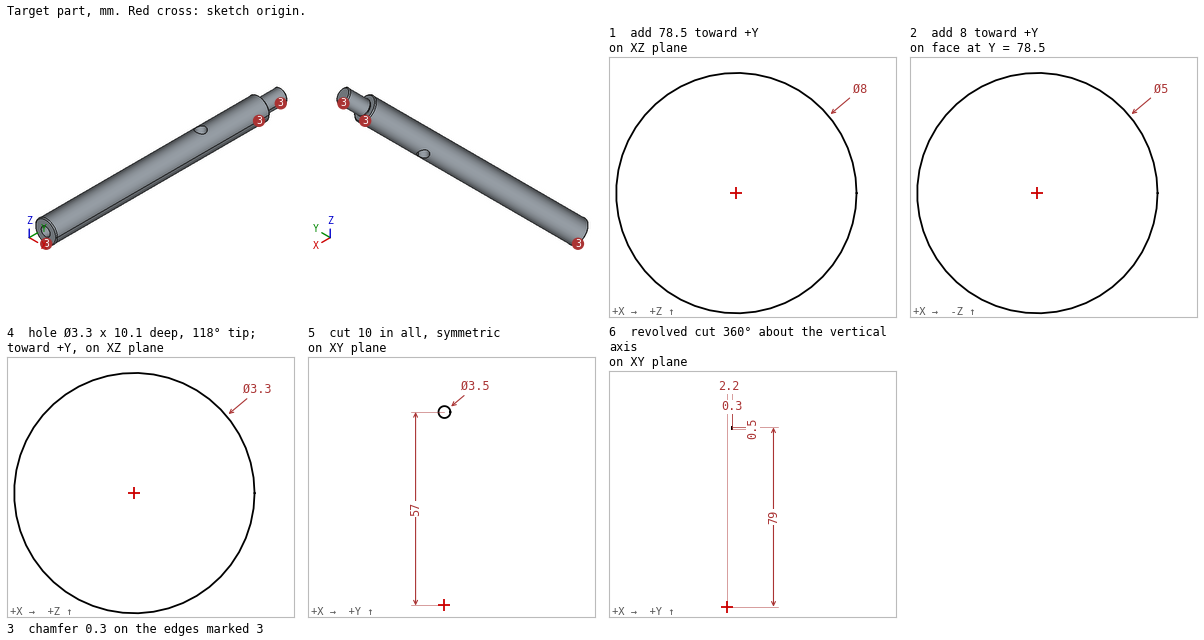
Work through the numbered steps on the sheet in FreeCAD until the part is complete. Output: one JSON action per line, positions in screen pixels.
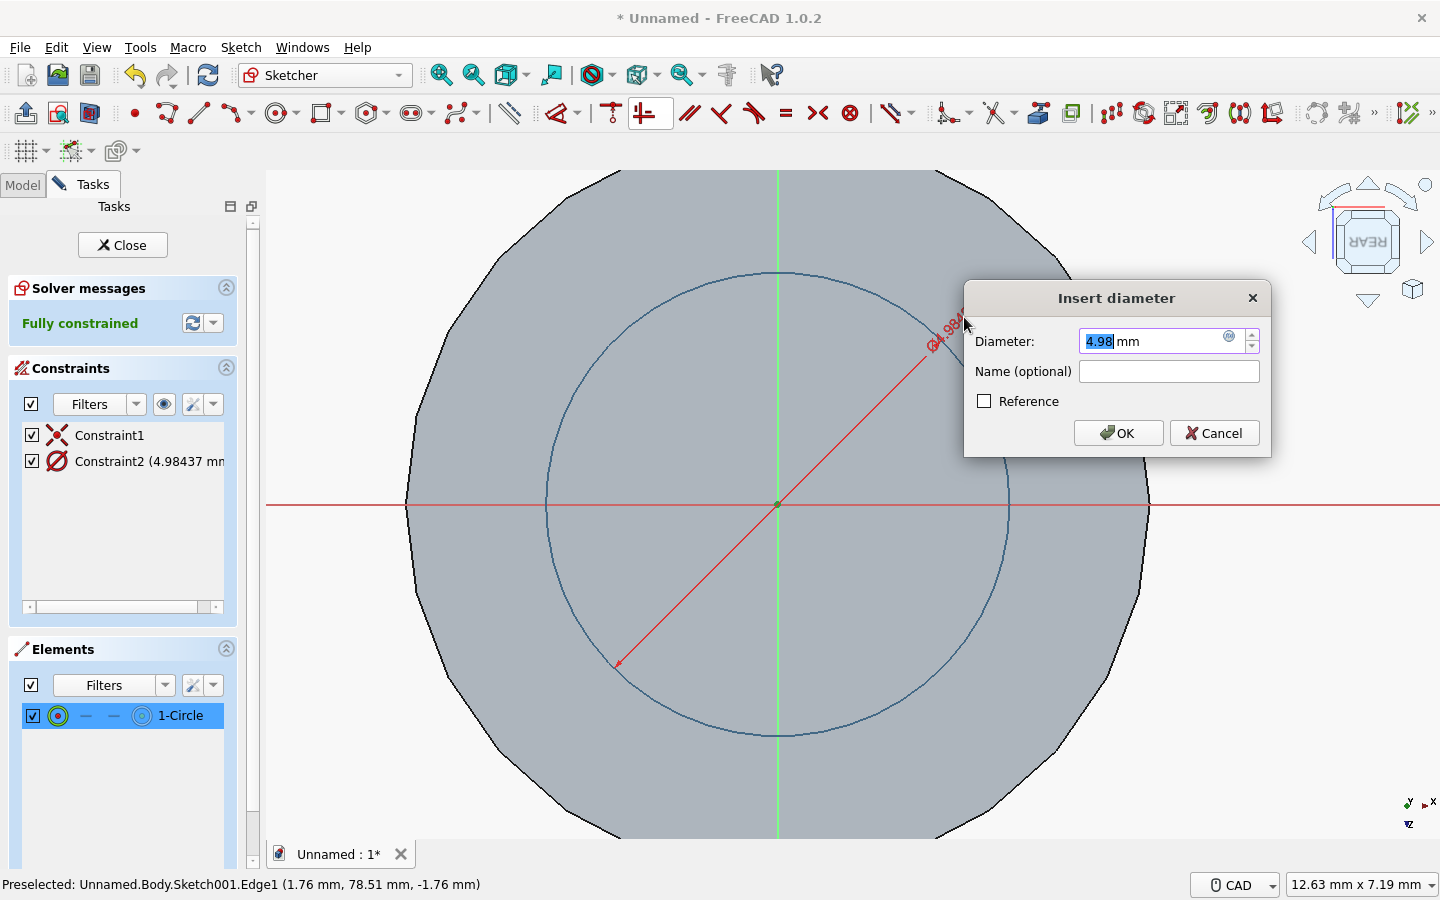
{"action": "type", "text": "5"}
{"action": "key", "text": "Return"}
{"action": "key", "text": "Escape"}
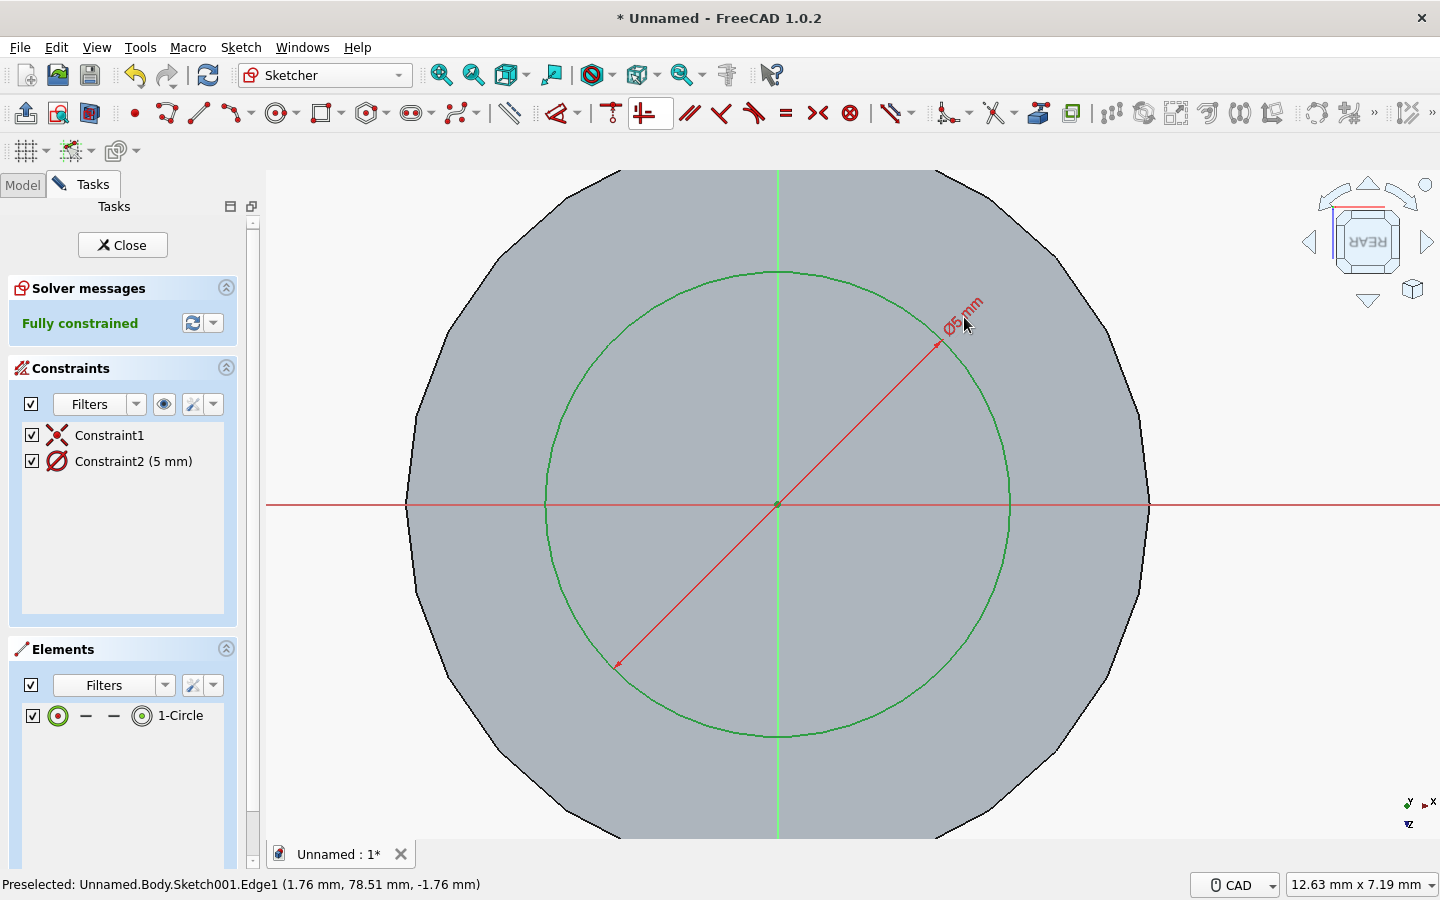
{"action": "left_click", "coordinate": [123, 245]}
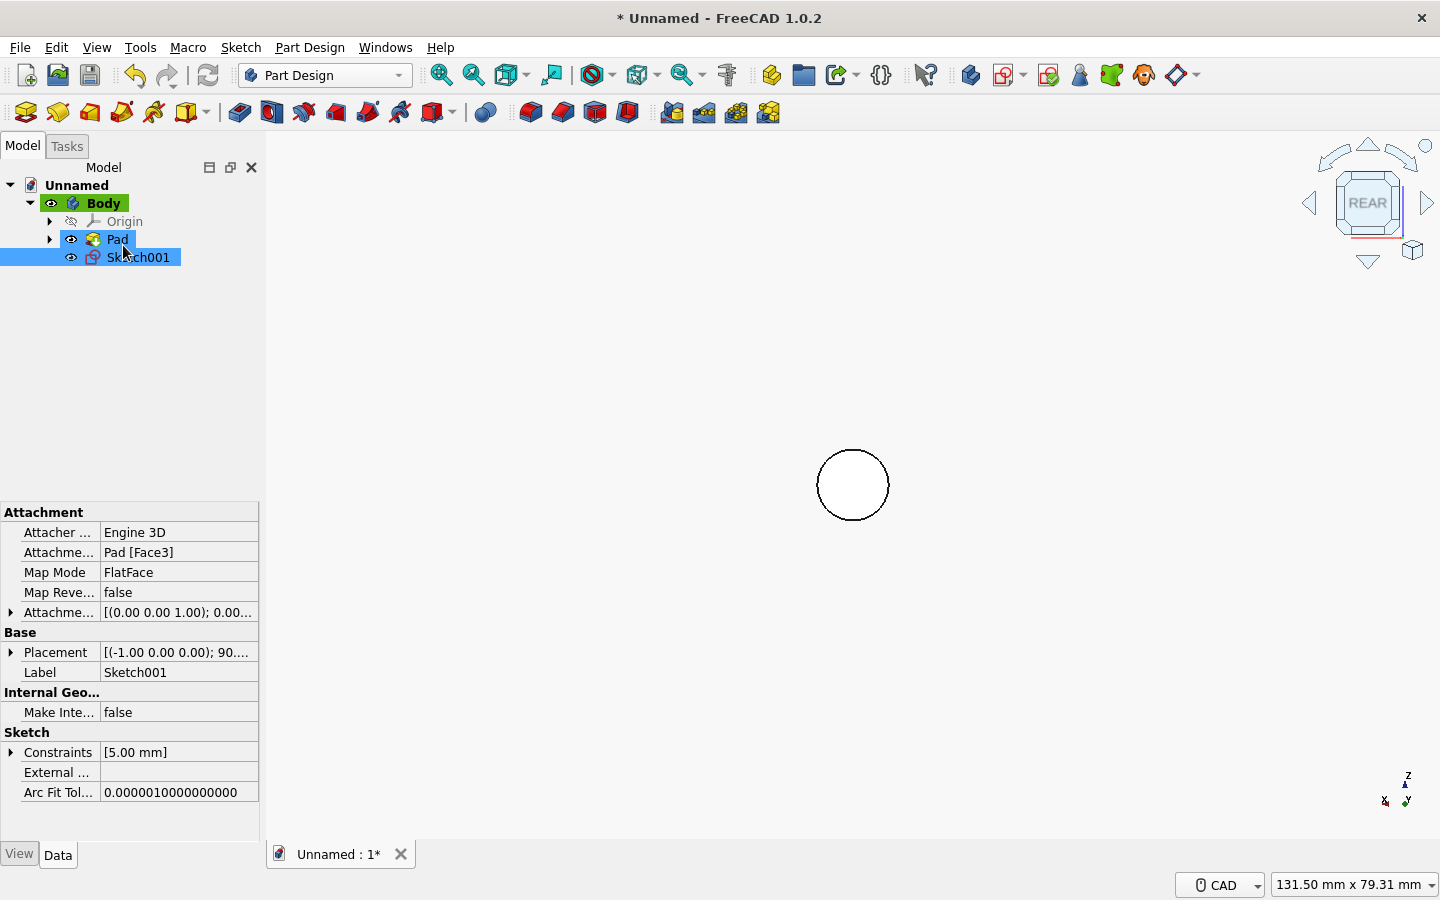
{"action": "left_click", "coordinate": [26, 112]}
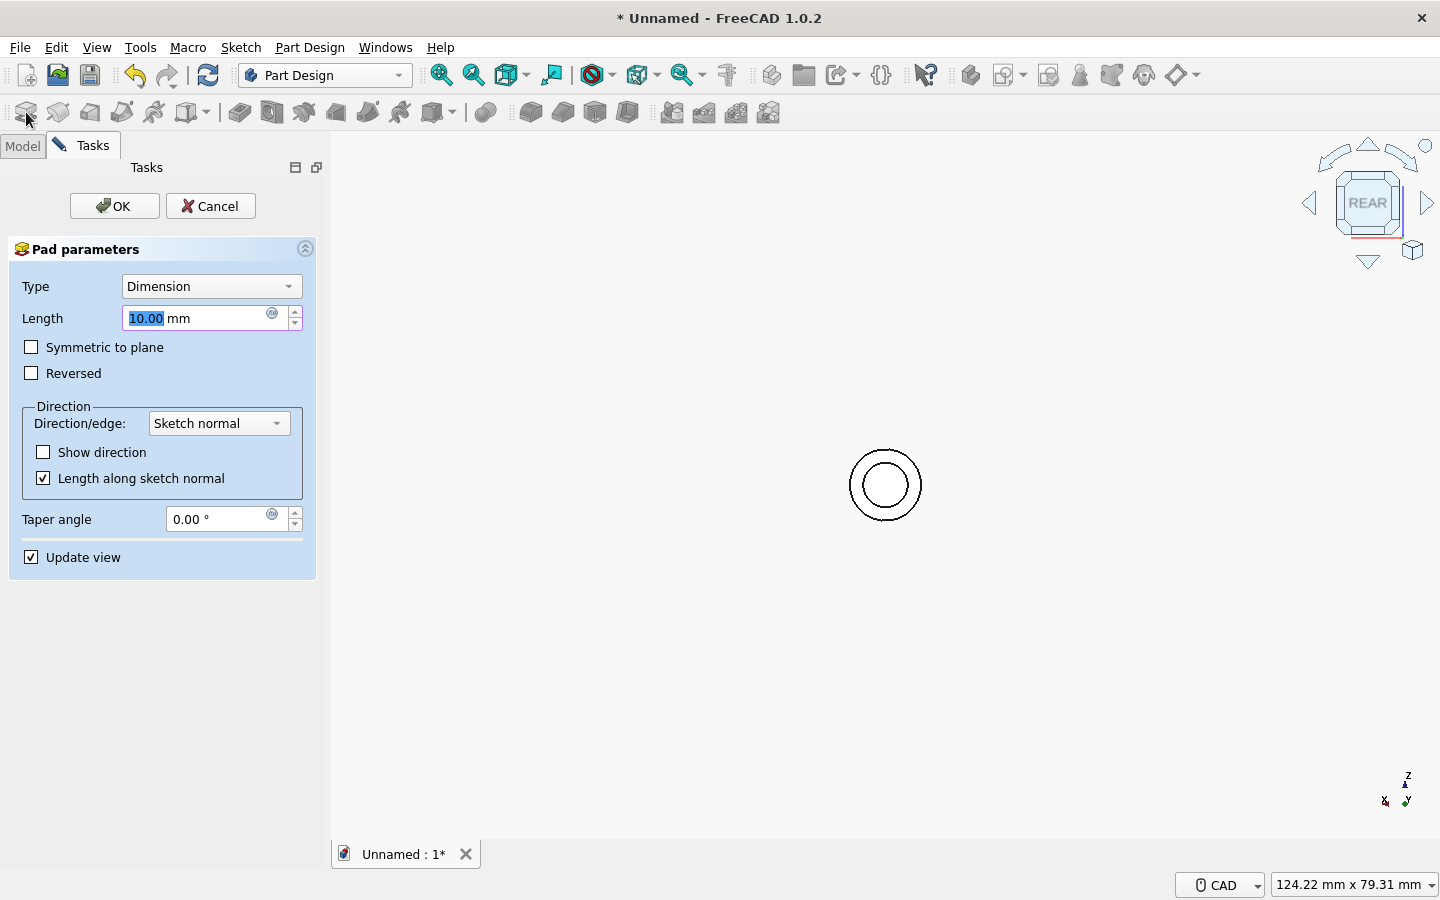
{"action": "type", "text": "8"}
{"action": "key", "text": "Tab"}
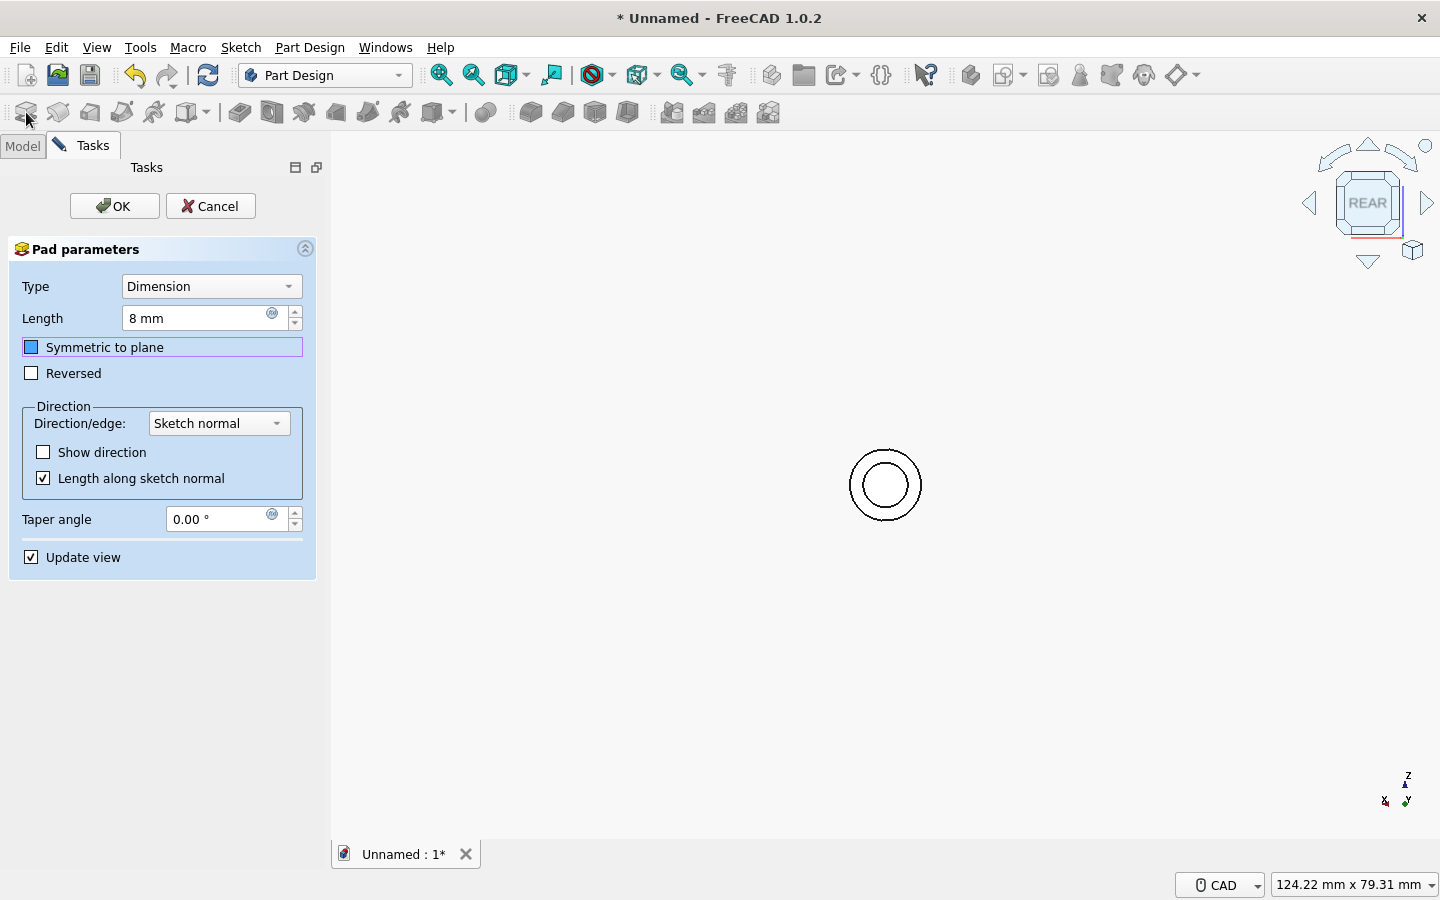
{"action": "left_click", "coordinate": [115, 206]}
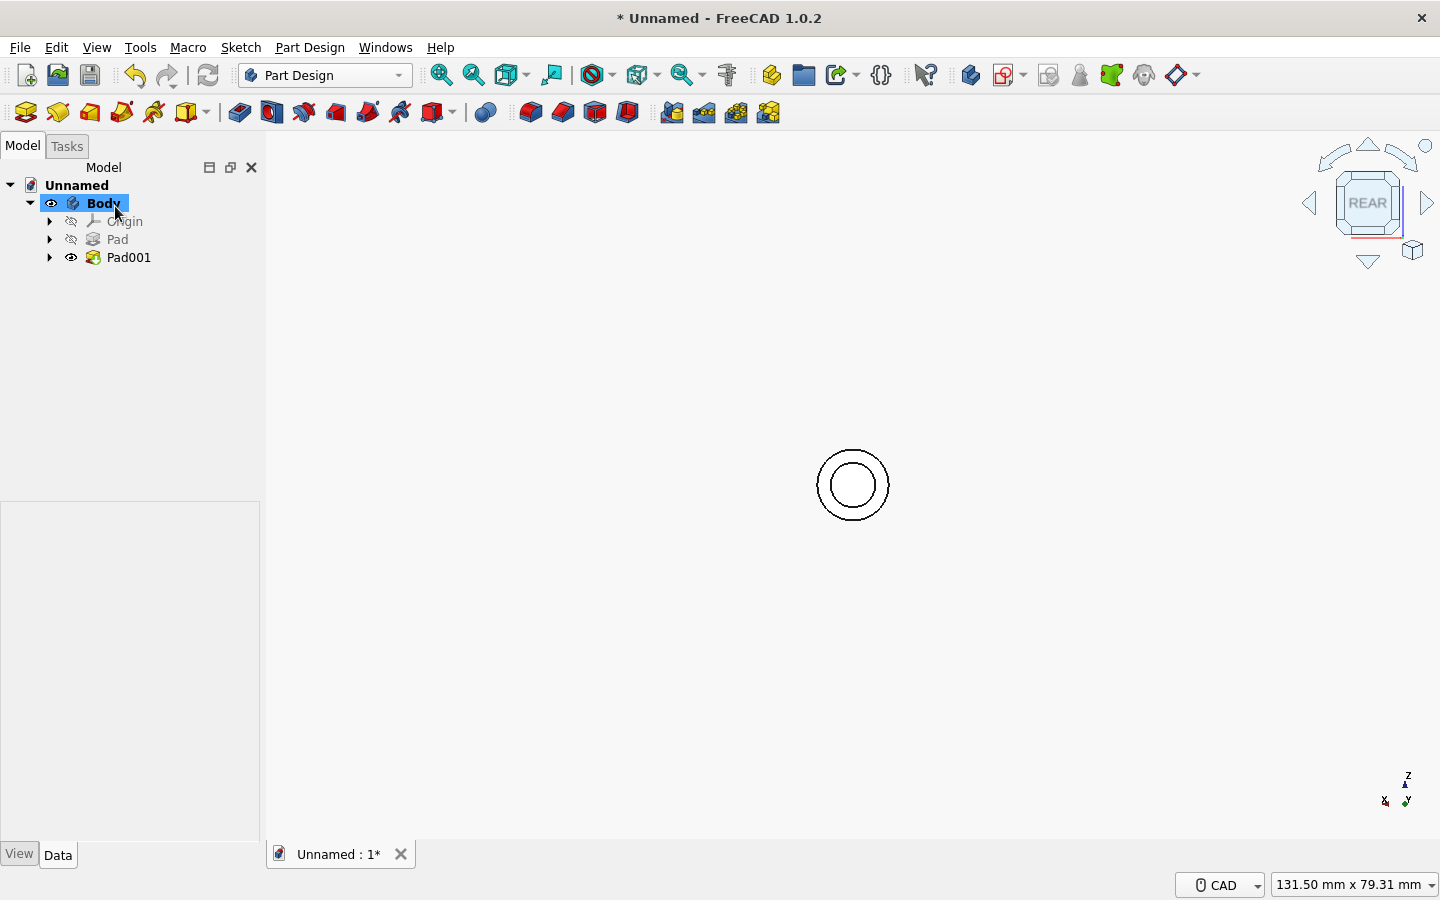
{"action": "left_click", "coordinate": [442, 76]}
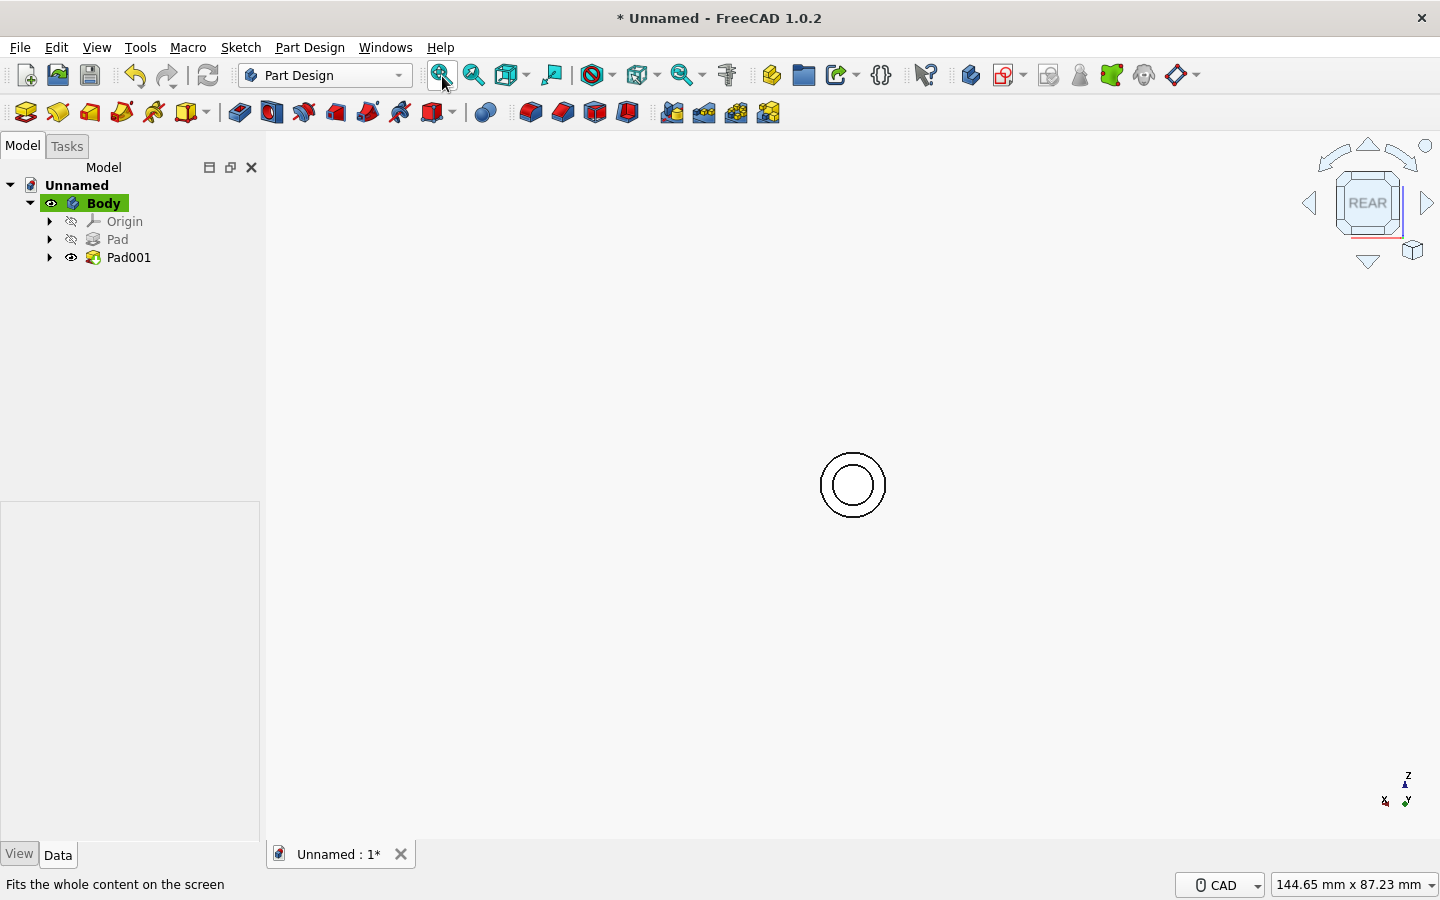
{"action": "left_click", "coordinate": [885, 484]}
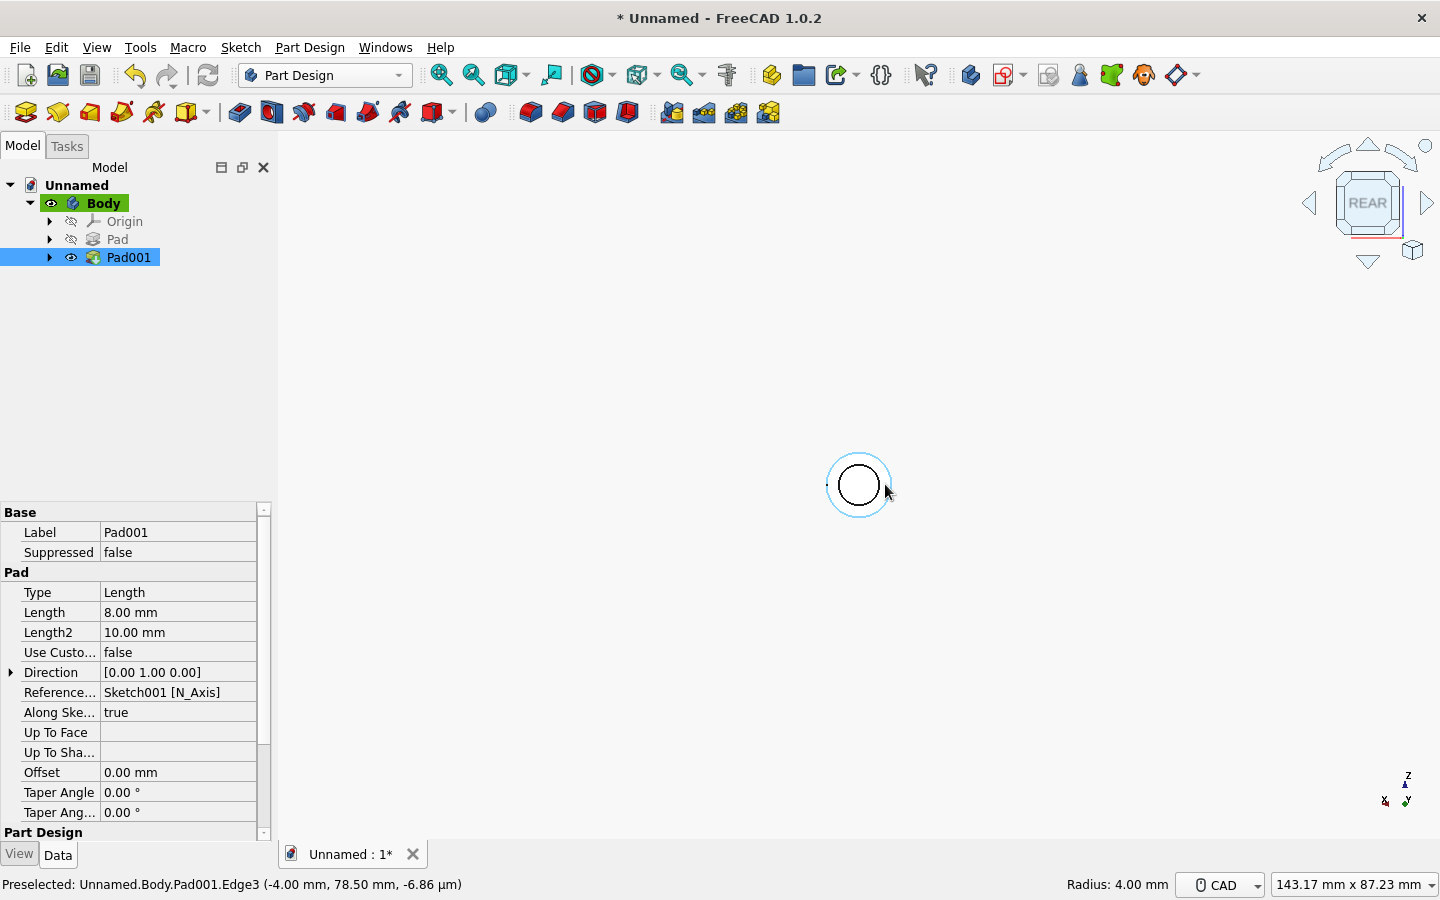
{"action": "left_click", "coordinate": [879, 484], "text": "ctrl"}